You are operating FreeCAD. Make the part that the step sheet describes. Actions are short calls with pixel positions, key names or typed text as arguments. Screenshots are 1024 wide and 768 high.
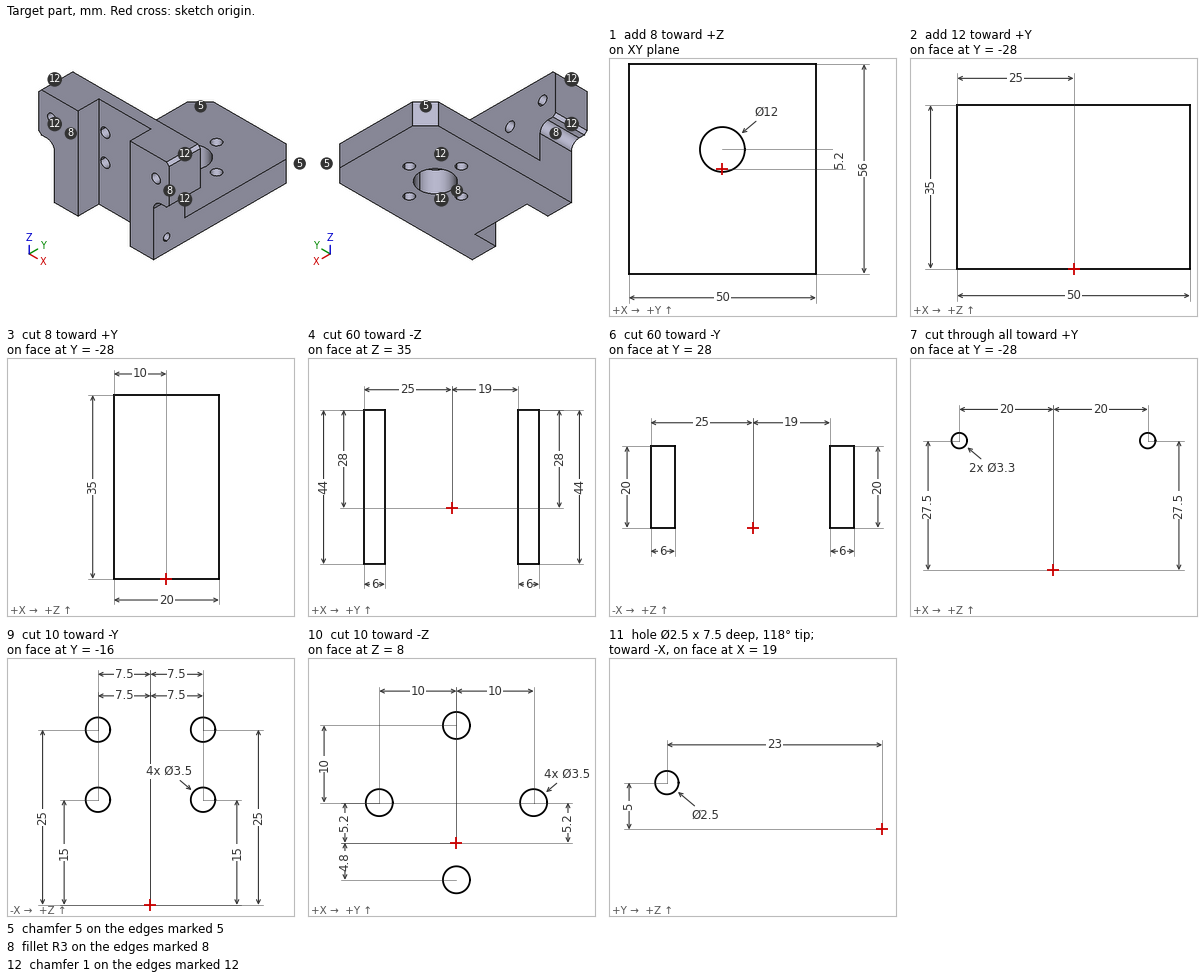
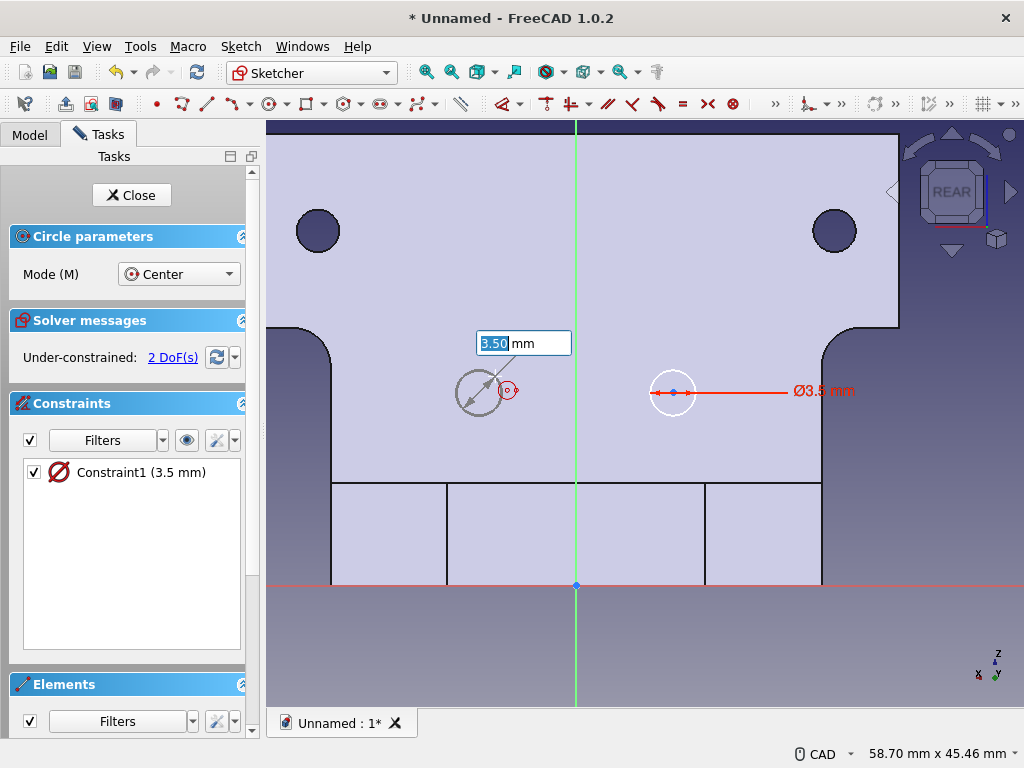
text(3.5)
key(Return)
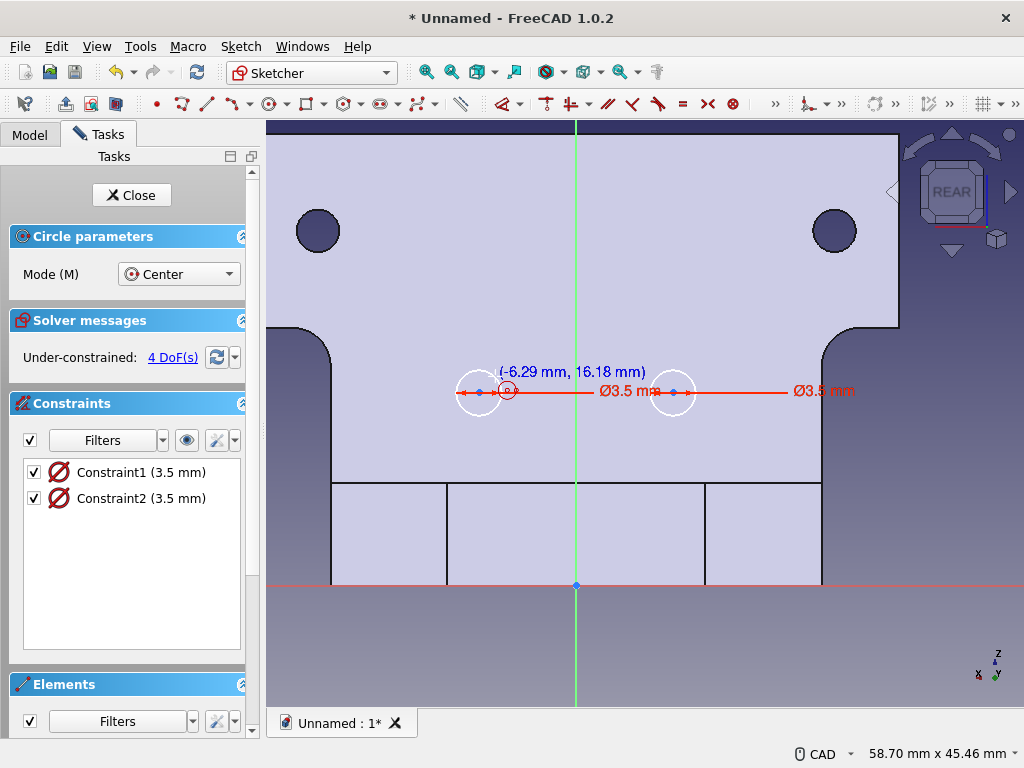
click(673, 263)
move(689, 247)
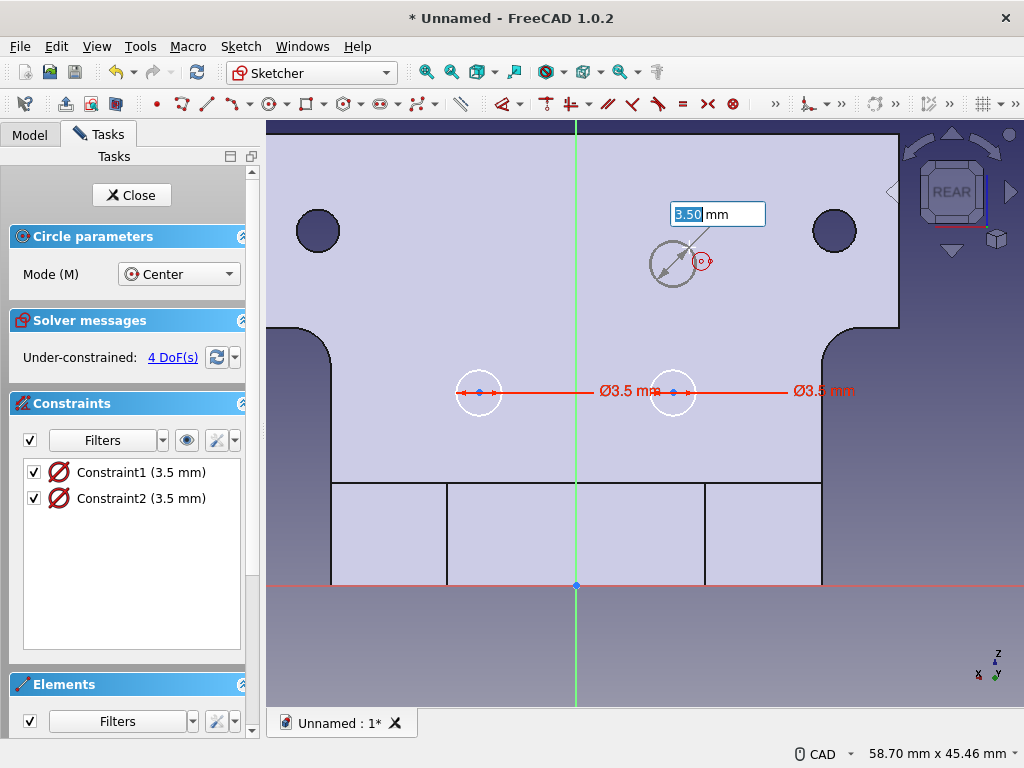
text(3.5)
key(Return)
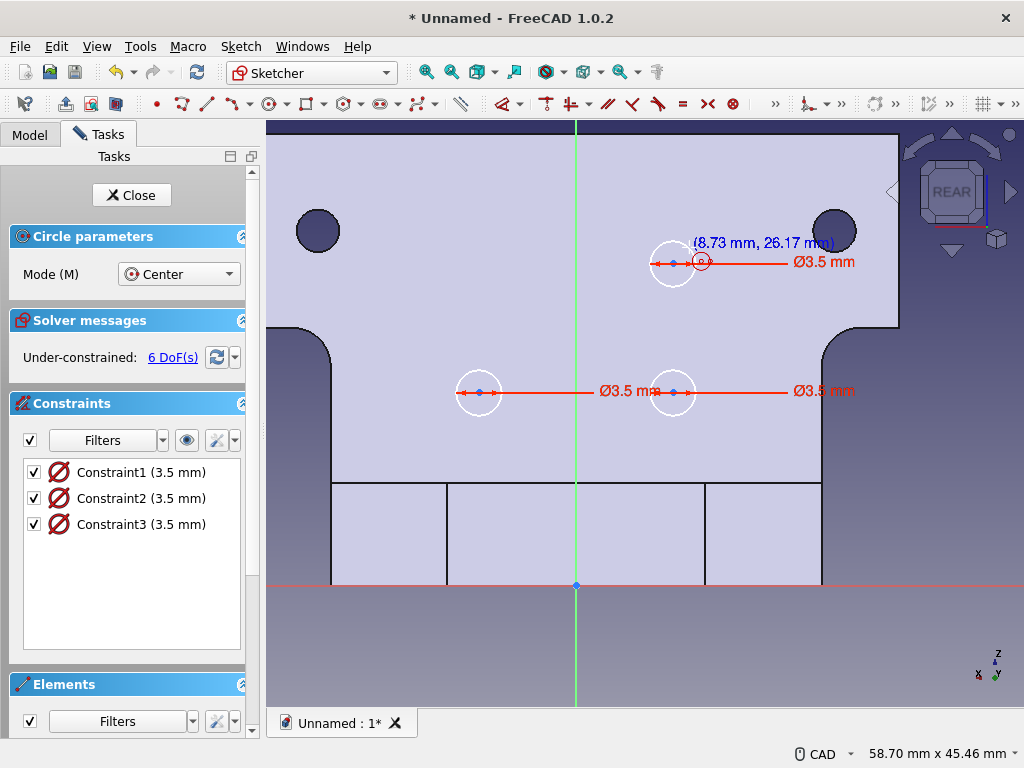
click(479, 263)
move(495, 247)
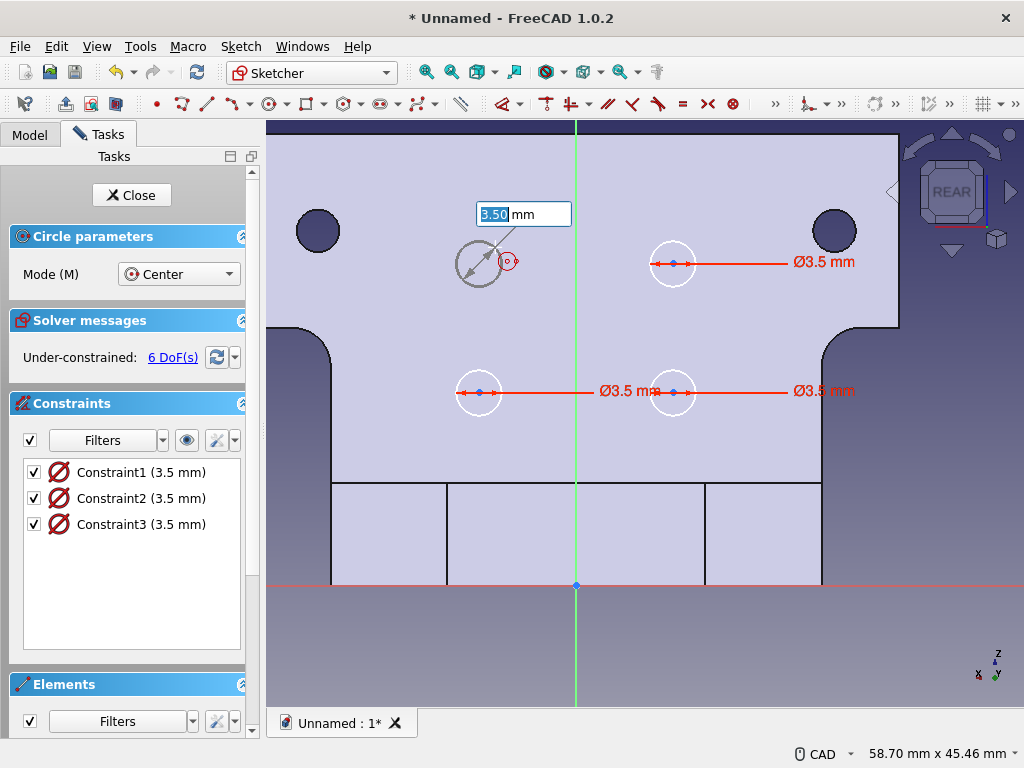
text(3.5)
key(Return)
key(Escape)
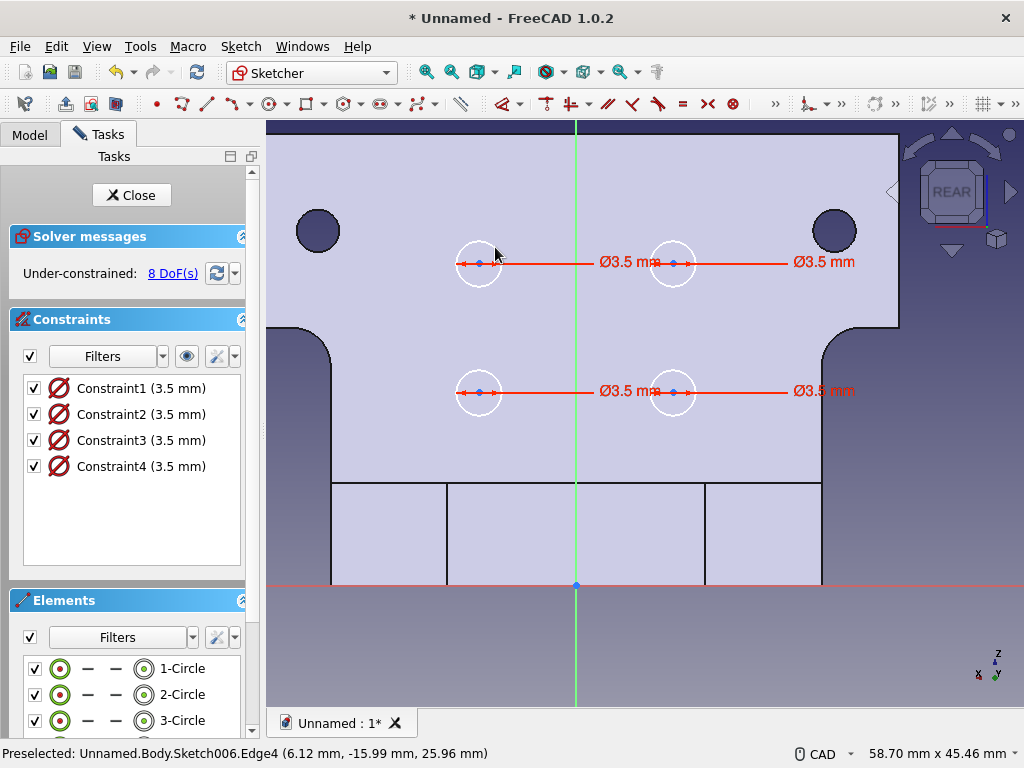
click(502, 104)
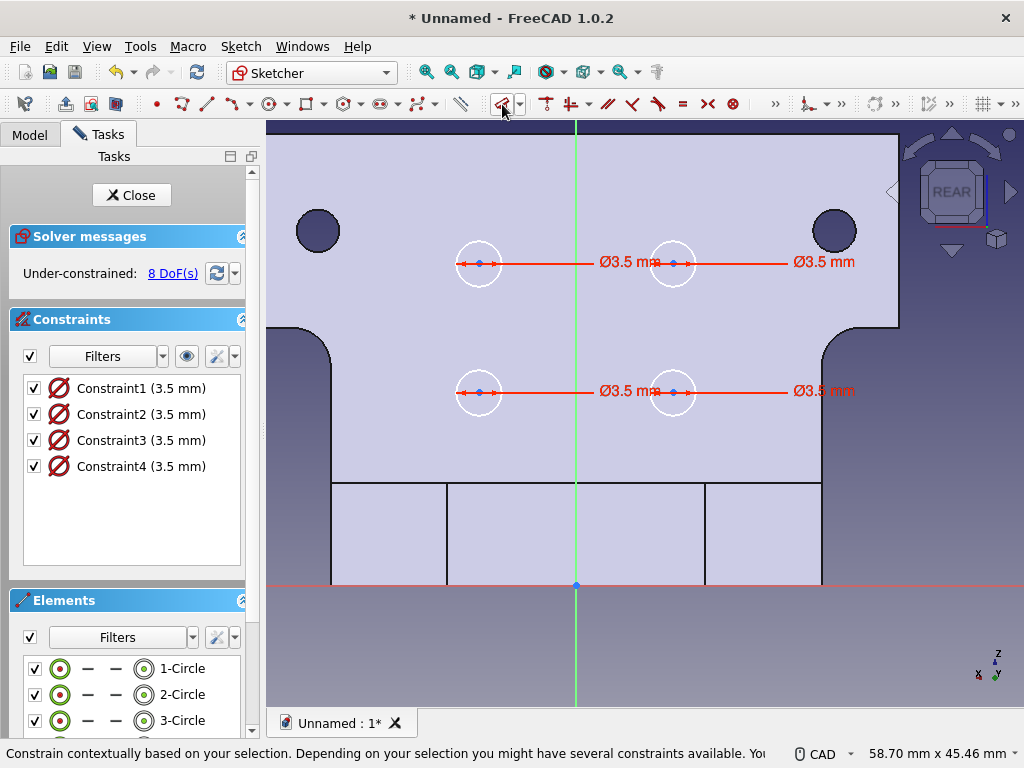
click(673, 393)
click(707, 489)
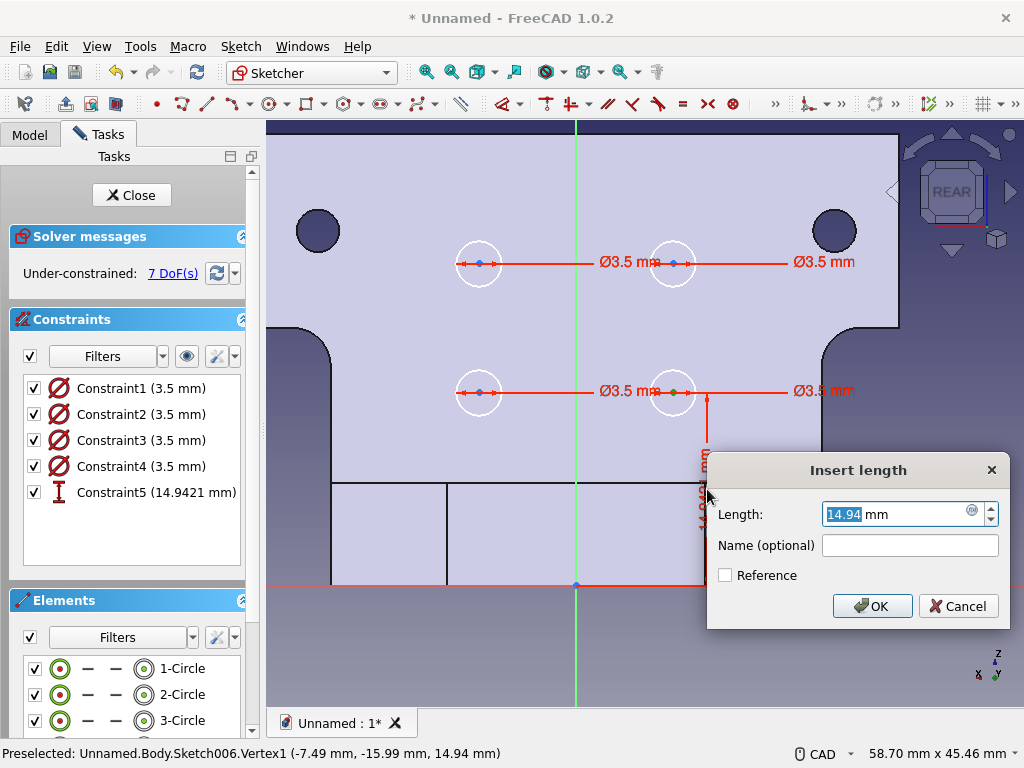
text(15)
key(Return)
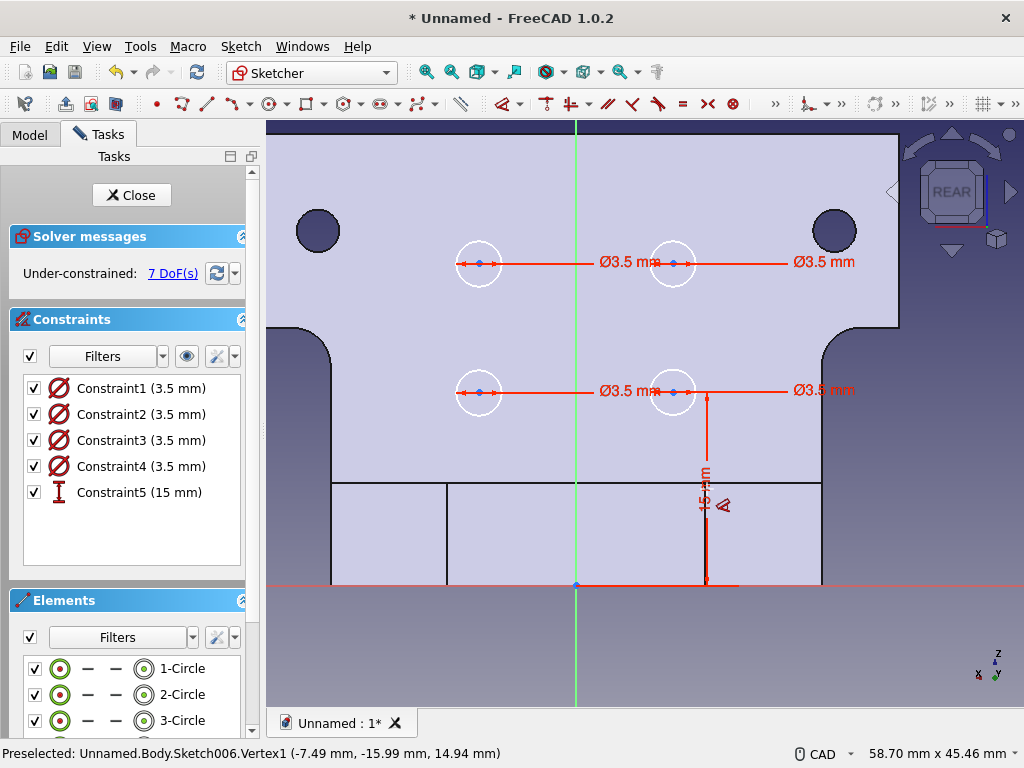
click(479, 393)
click(445, 489)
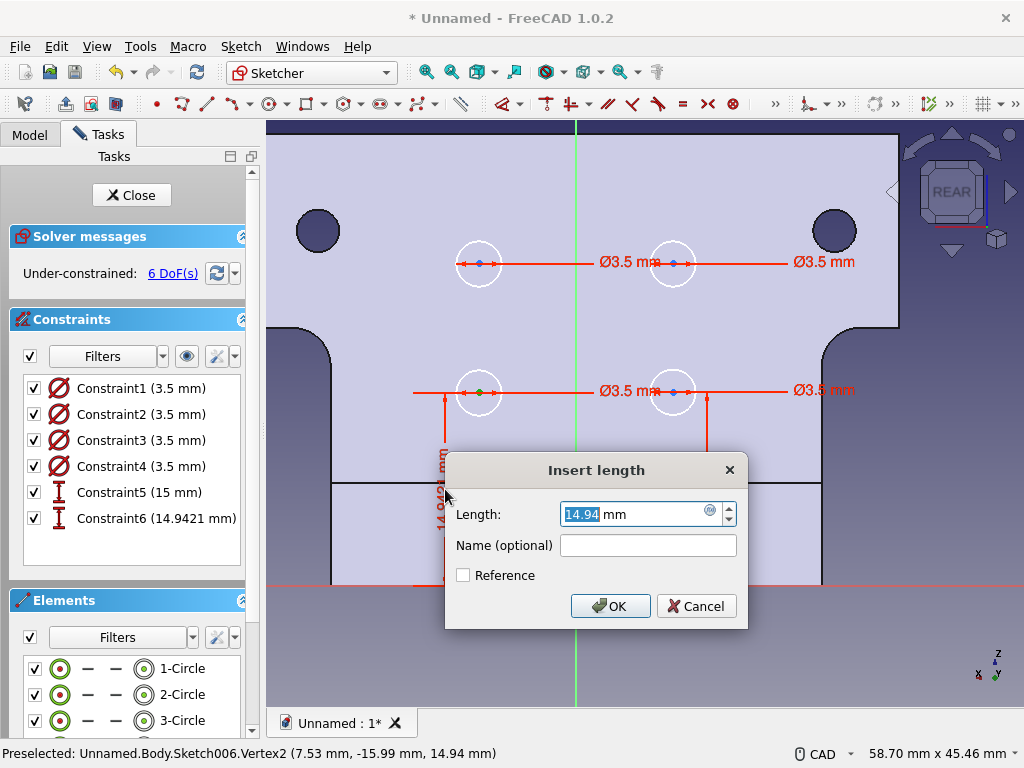
text(15)
key(Return)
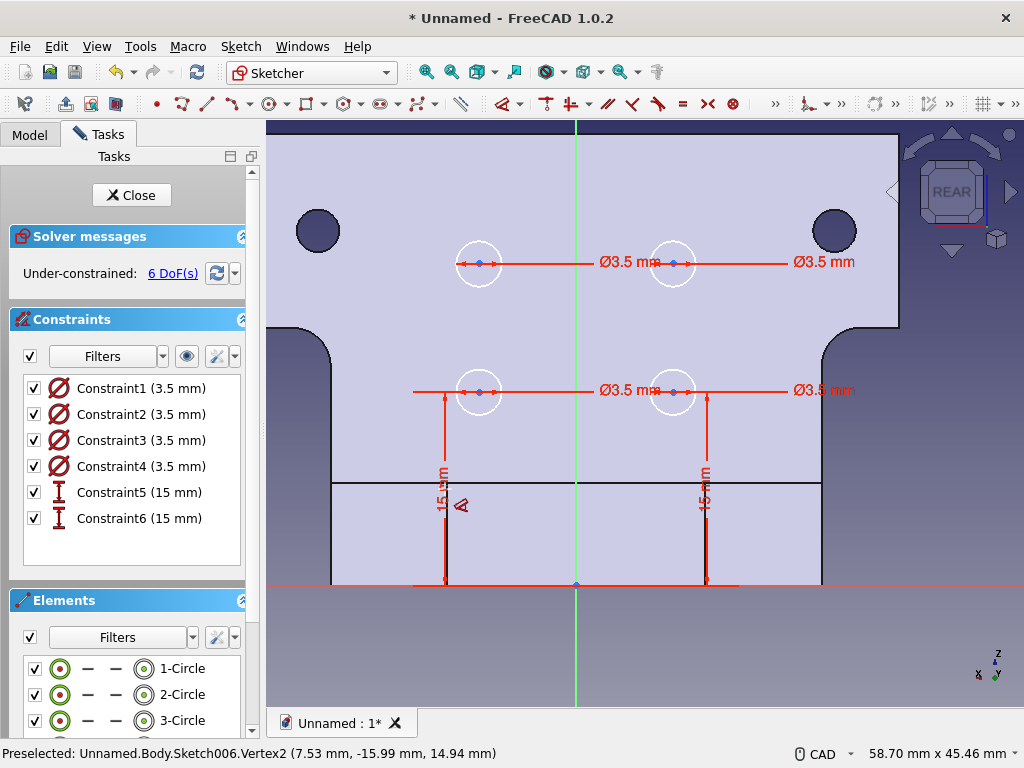
click(673, 264)
click(707, 425)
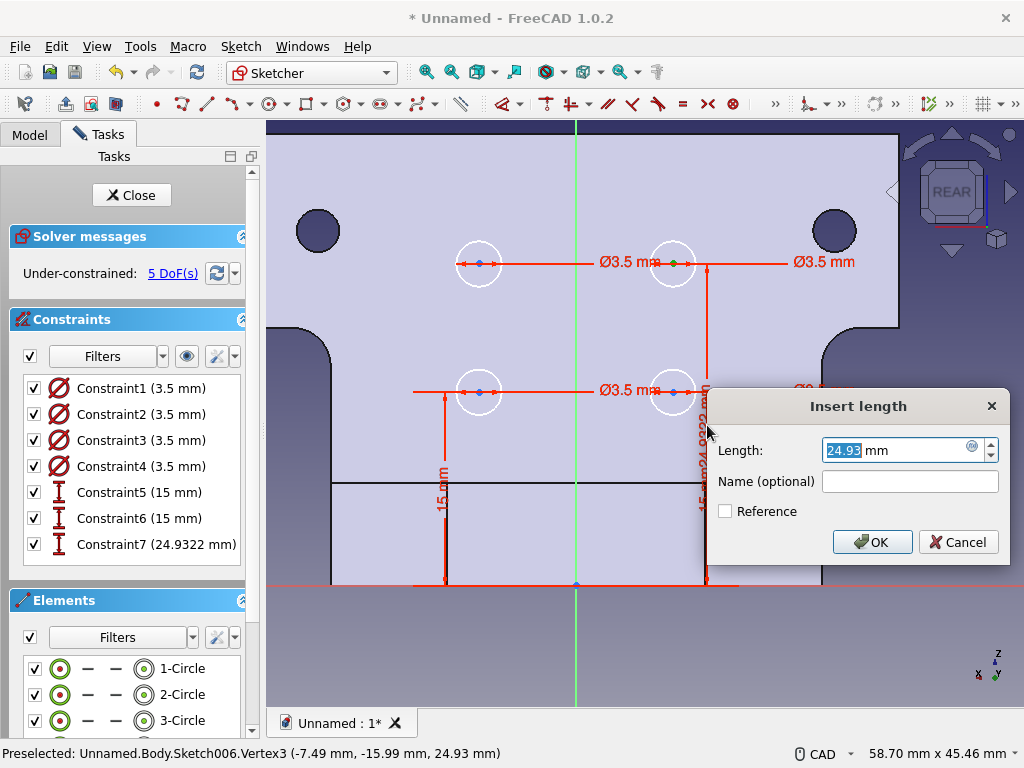
text(25)
key(Return)